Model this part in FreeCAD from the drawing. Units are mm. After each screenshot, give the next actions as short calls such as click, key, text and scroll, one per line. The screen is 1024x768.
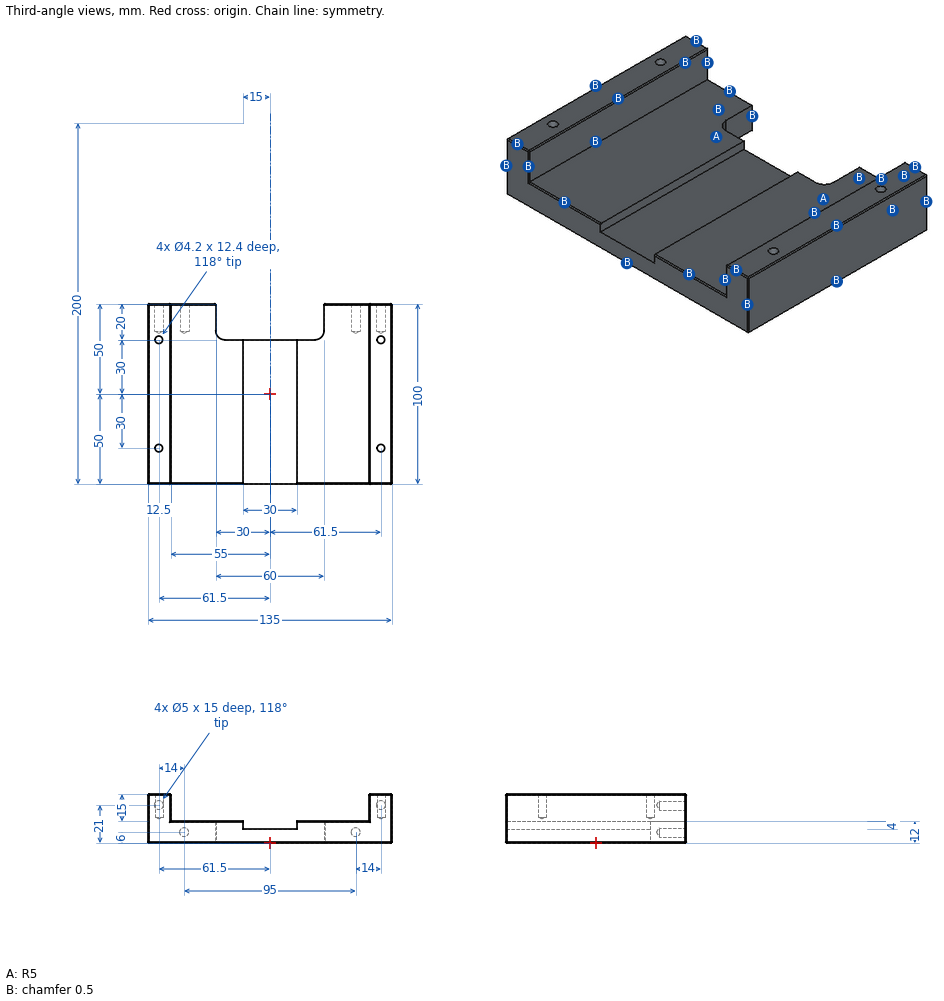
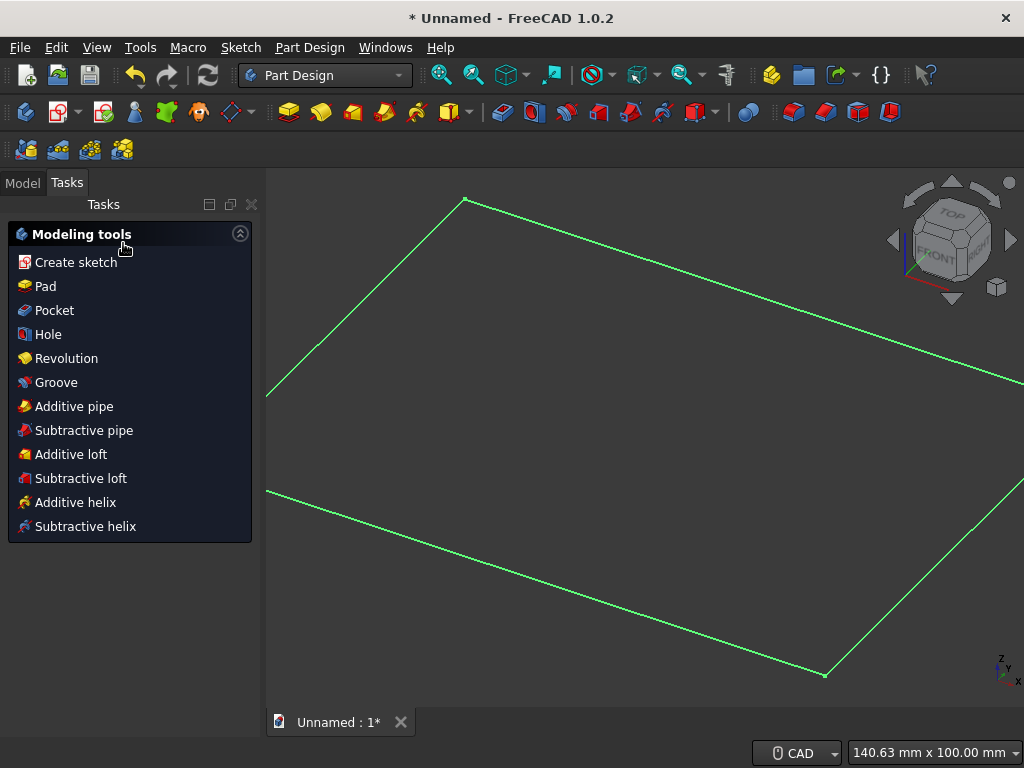
click(290, 112)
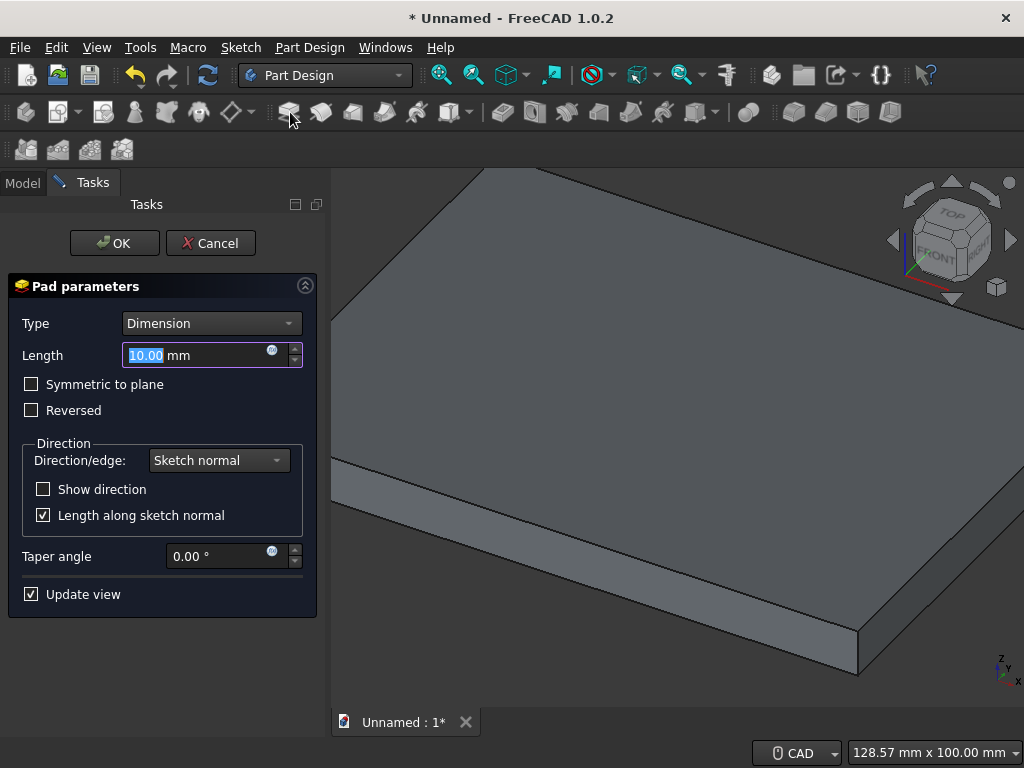
text(12)
key(Tab)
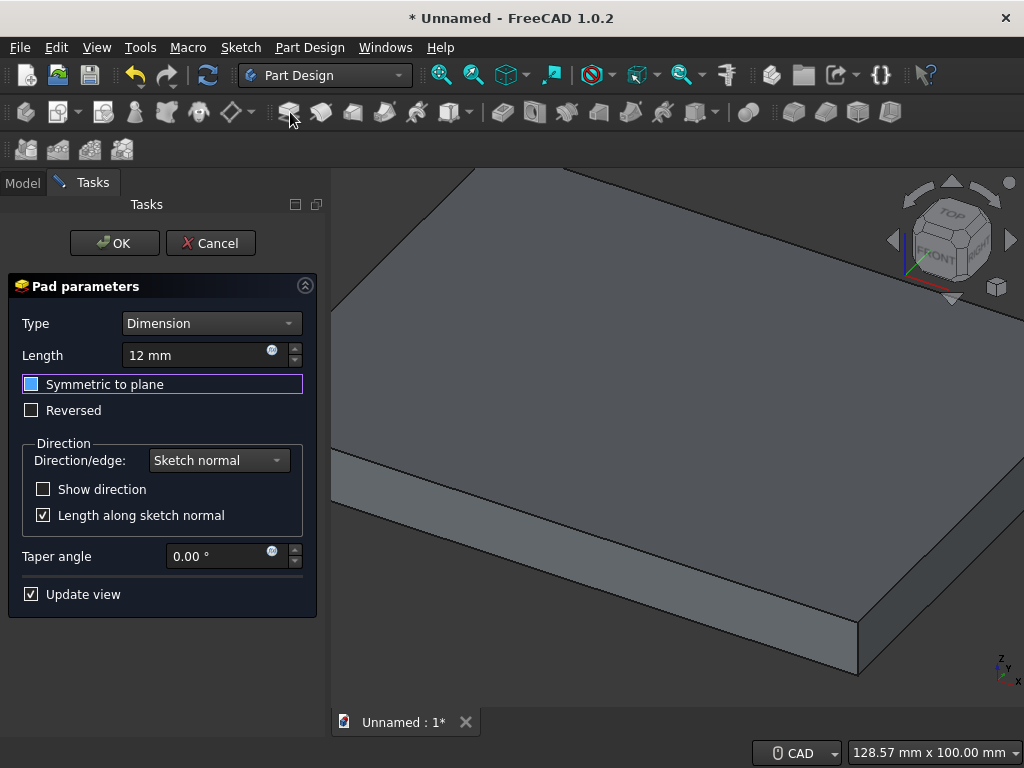
click(115, 243)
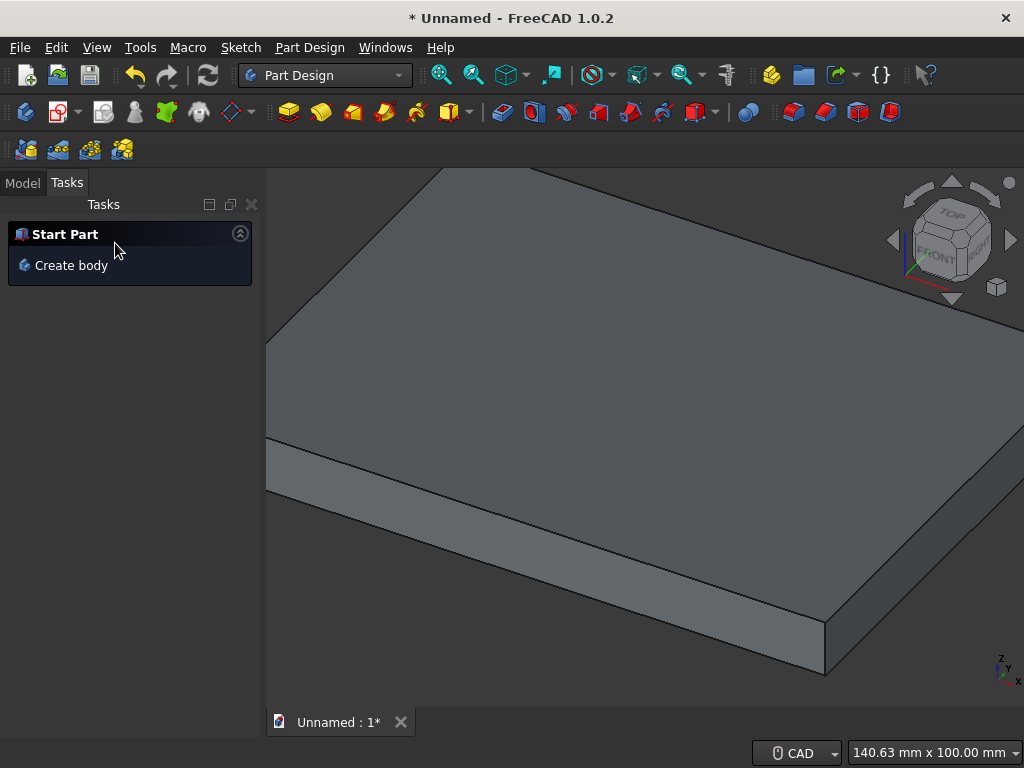
key(v)
key(f)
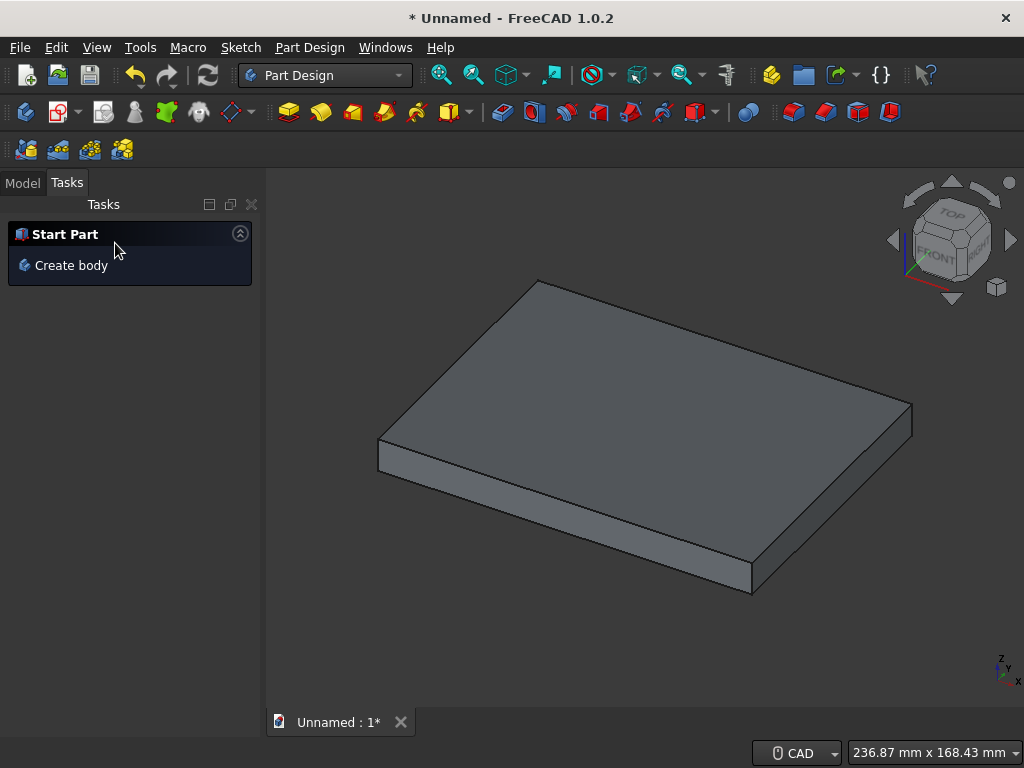
click(645, 421)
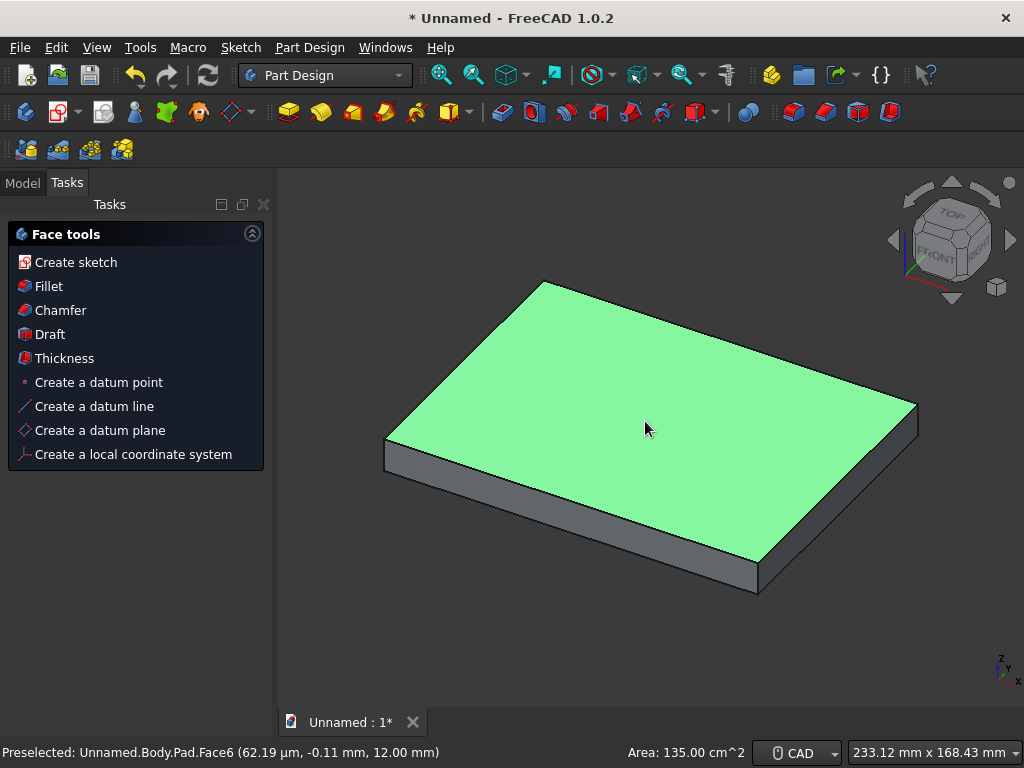
click(58, 112)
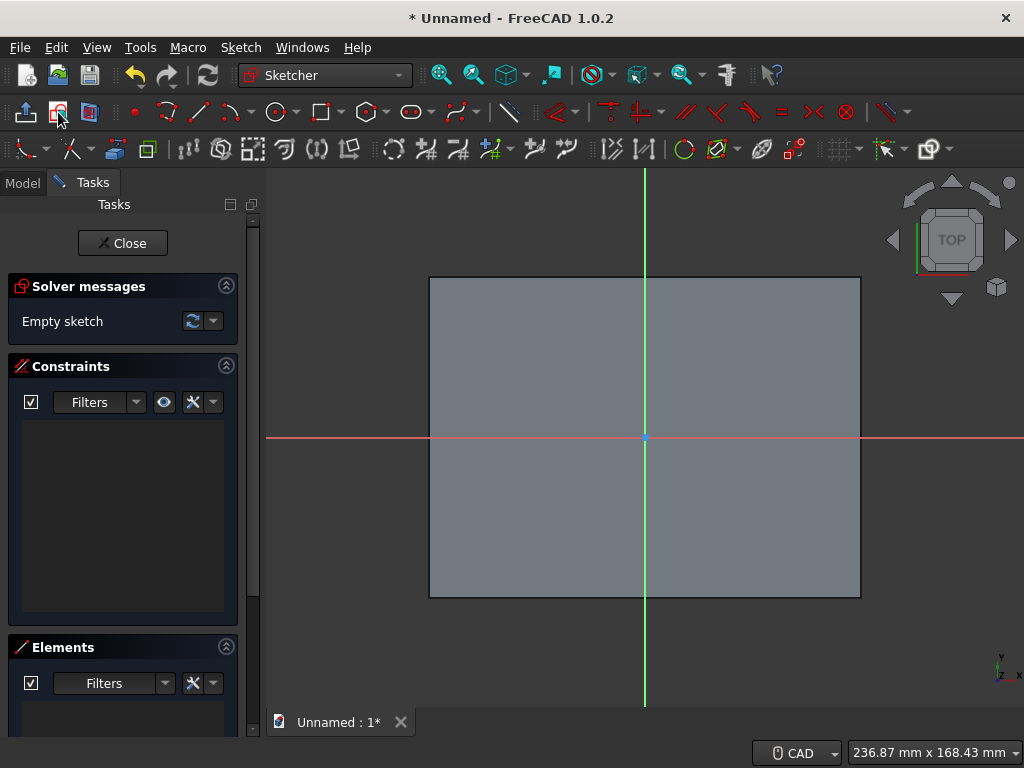
scroll(294, 437, down, 1)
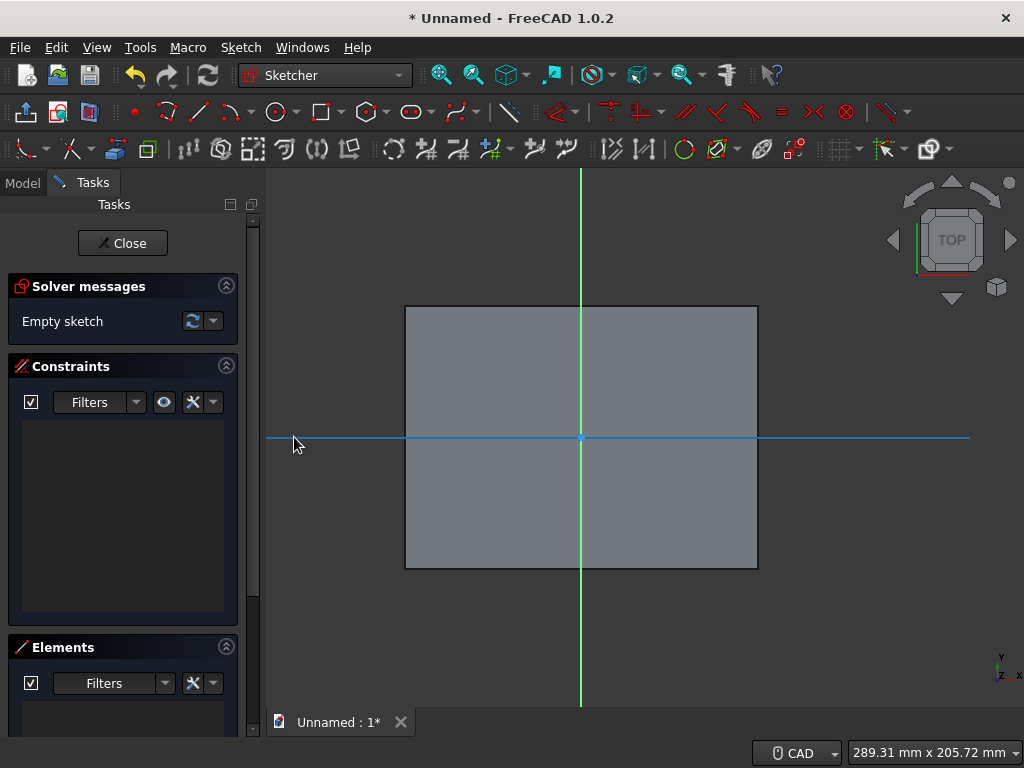
key(g)
key(r)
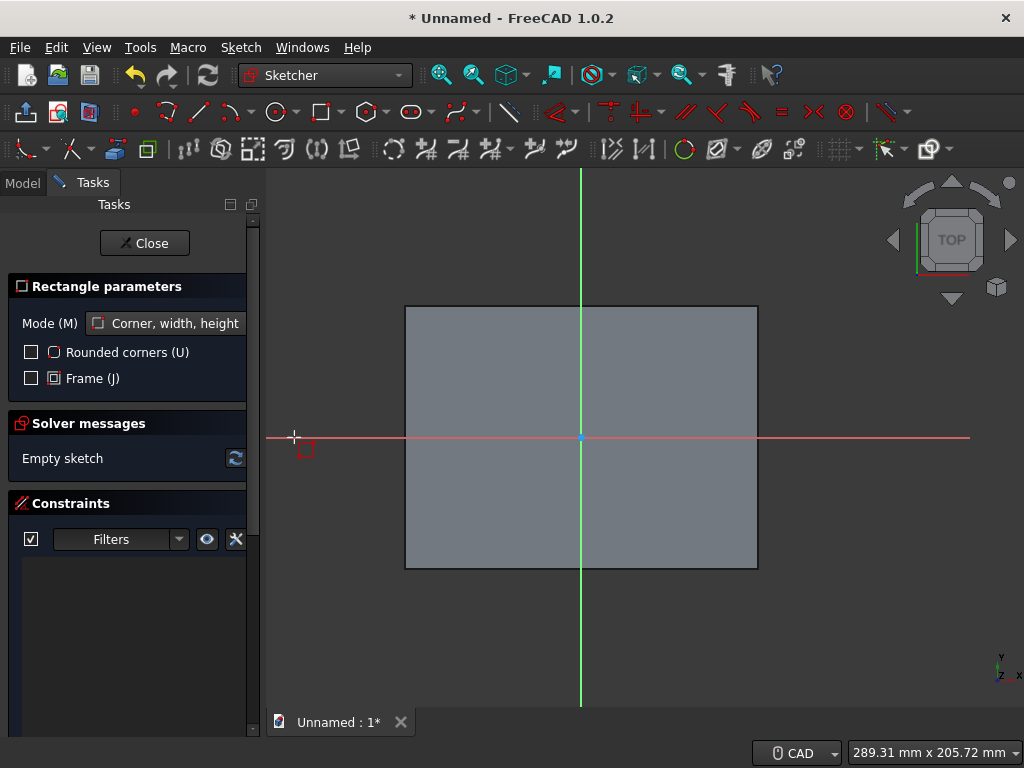
click(405, 306)
click(437, 569)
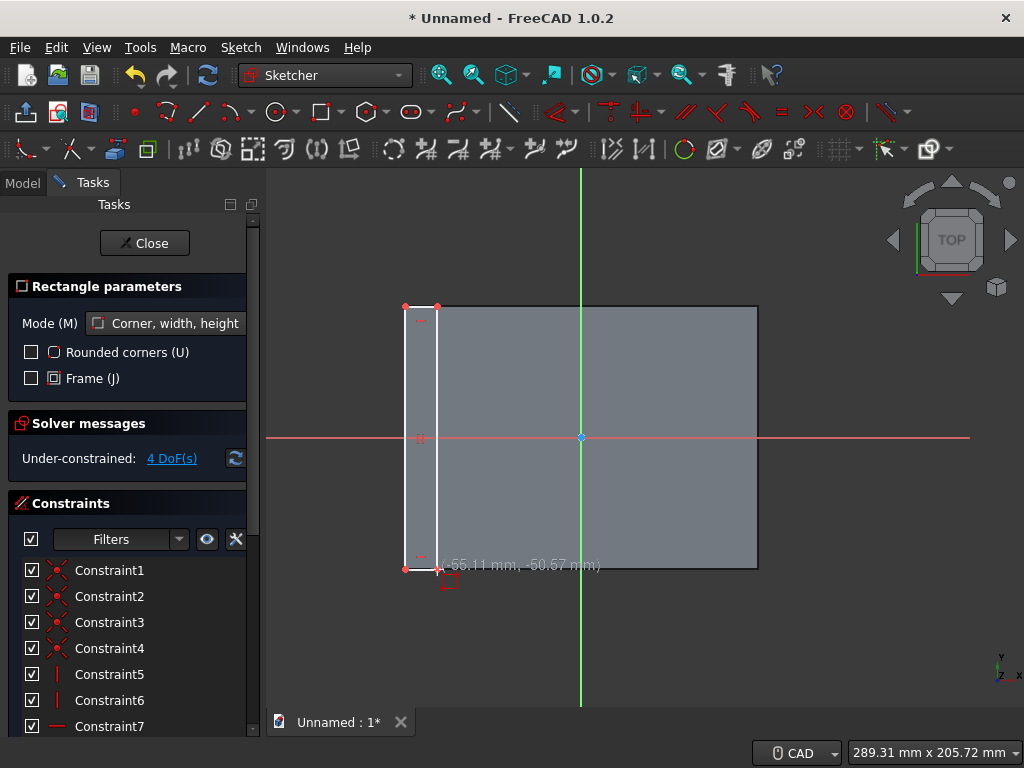
click(725, 306)
click(758, 569)
key(Escape)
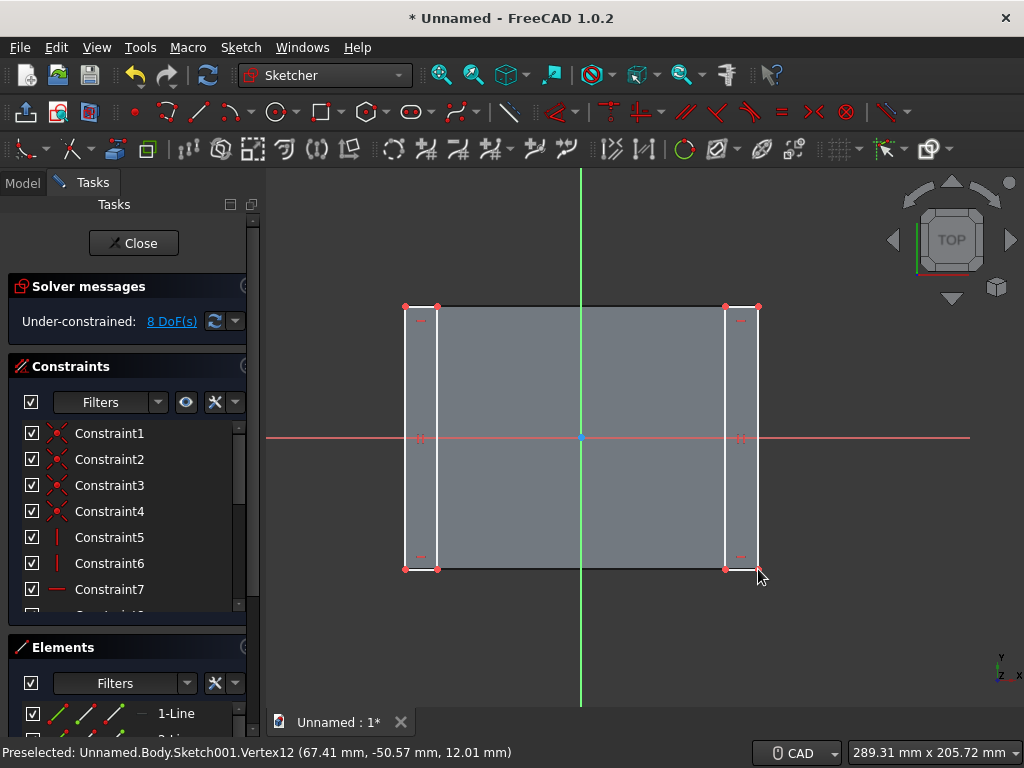
click(437, 307)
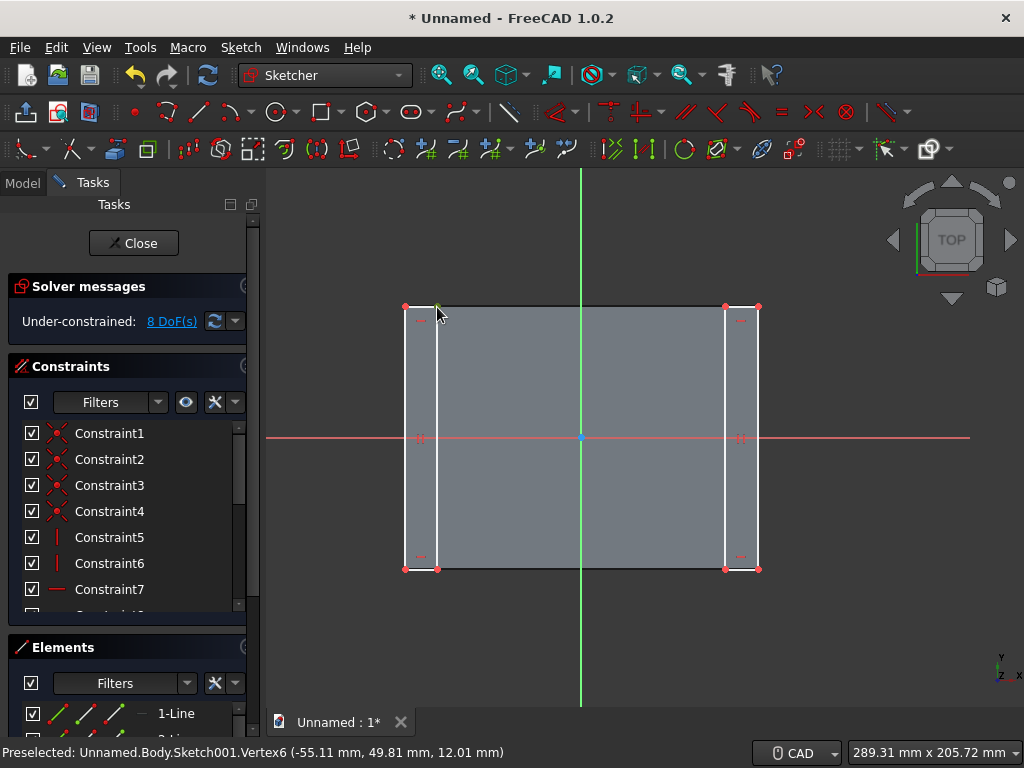
click(725, 307)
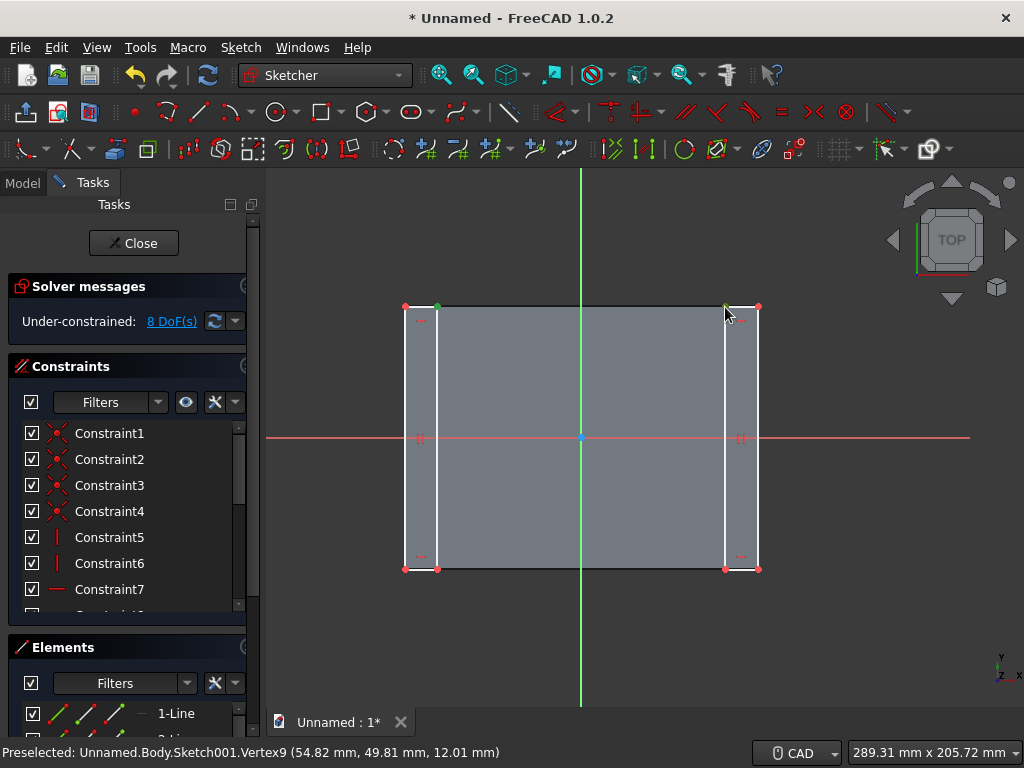
click(581, 644)